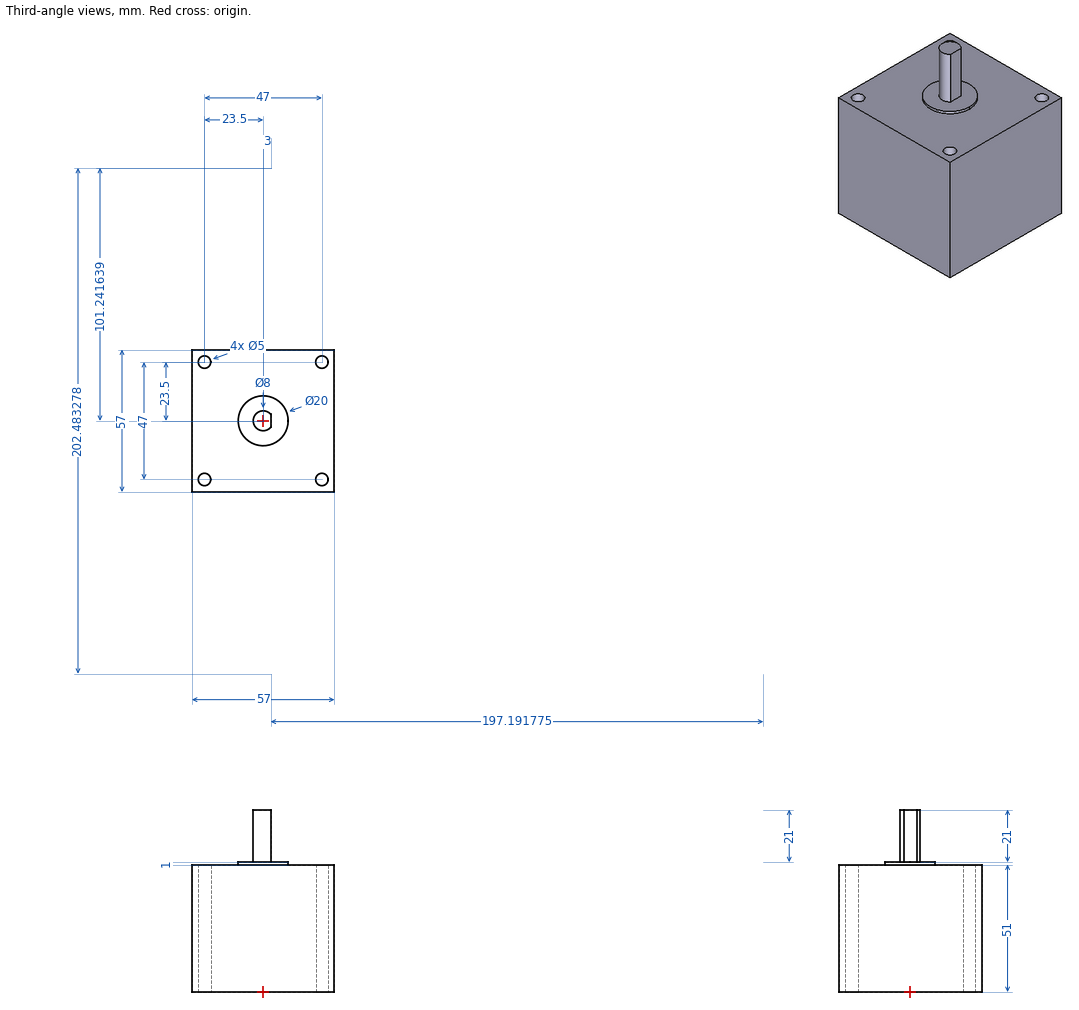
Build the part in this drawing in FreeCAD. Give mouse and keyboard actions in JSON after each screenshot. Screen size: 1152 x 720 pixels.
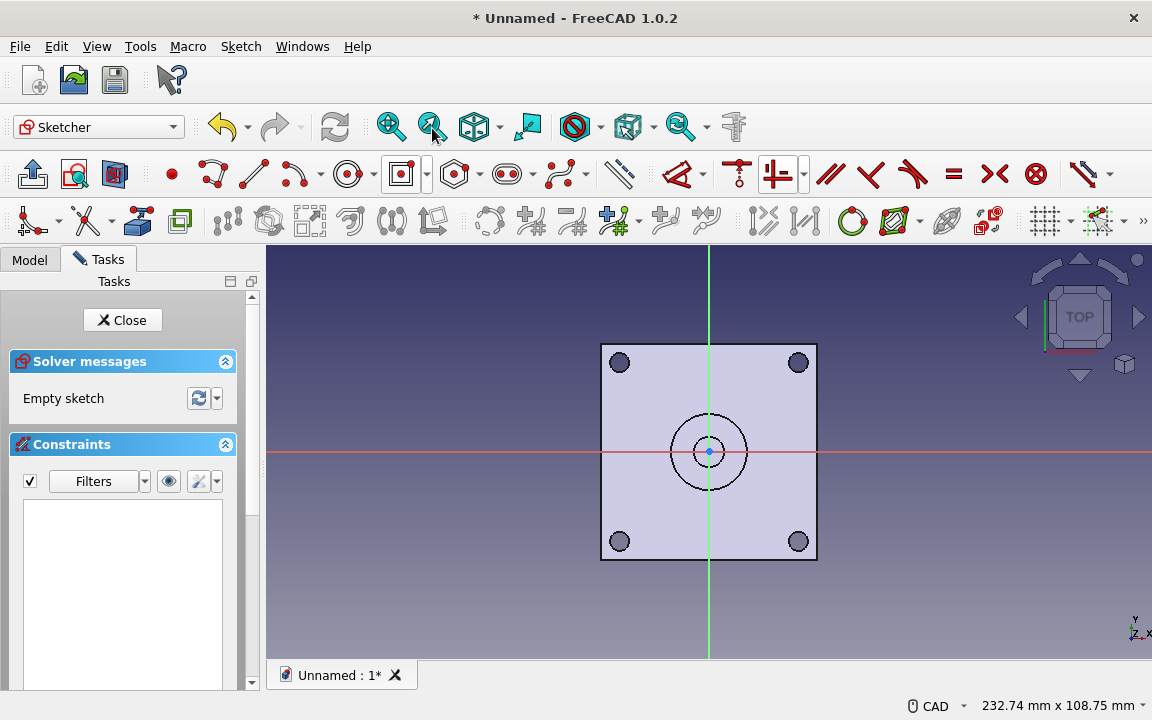
{"action": "scroll", "coordinate": [447, 452], "scroll_direction": "down", "scroll_amount": 6}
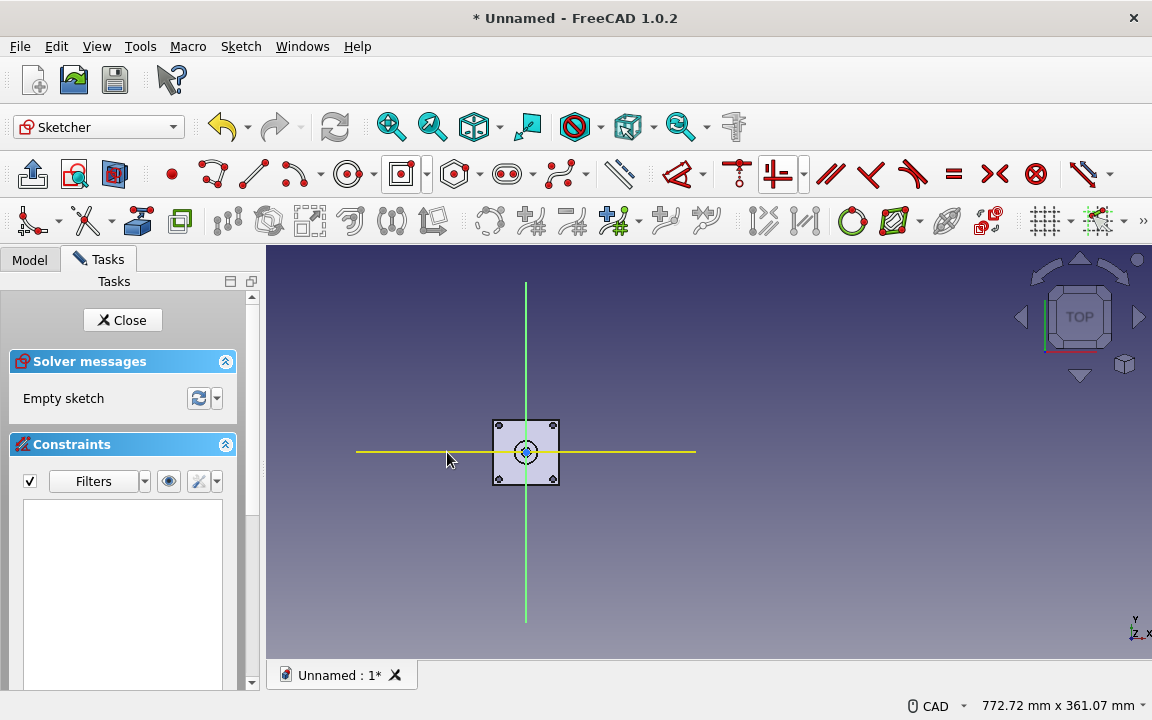
{"action": "left_click", "coordinate": [426, 174]}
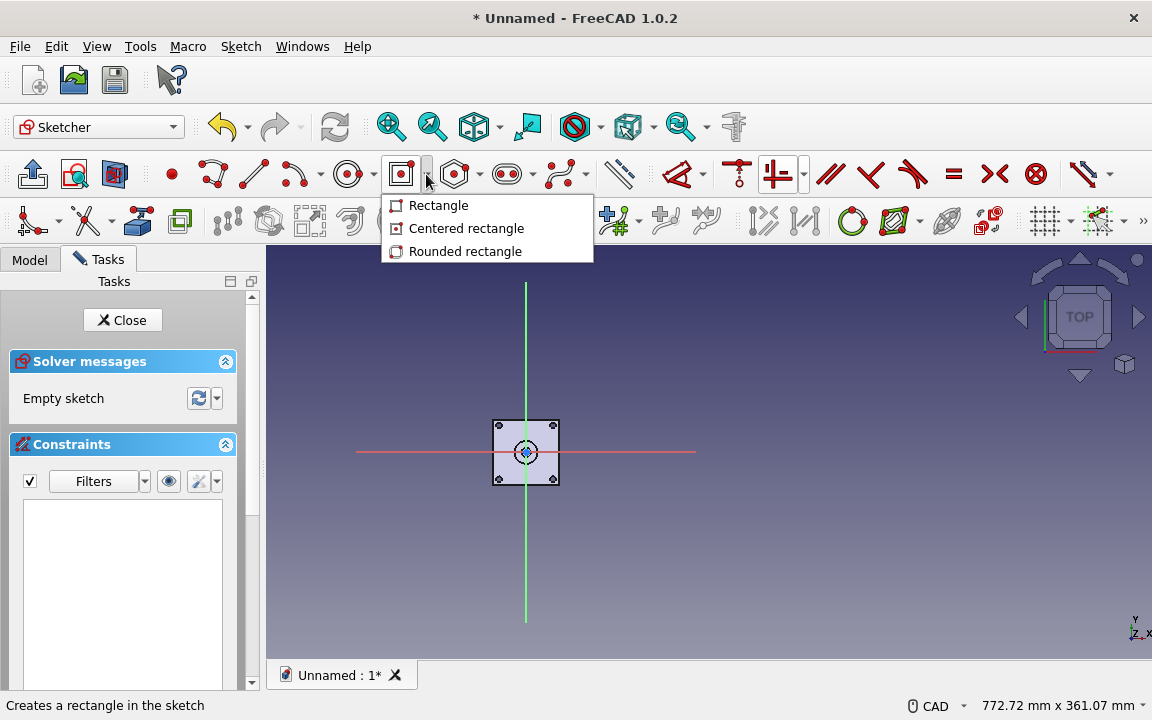
{"action": "left_click", "coordinate": [488, 206]}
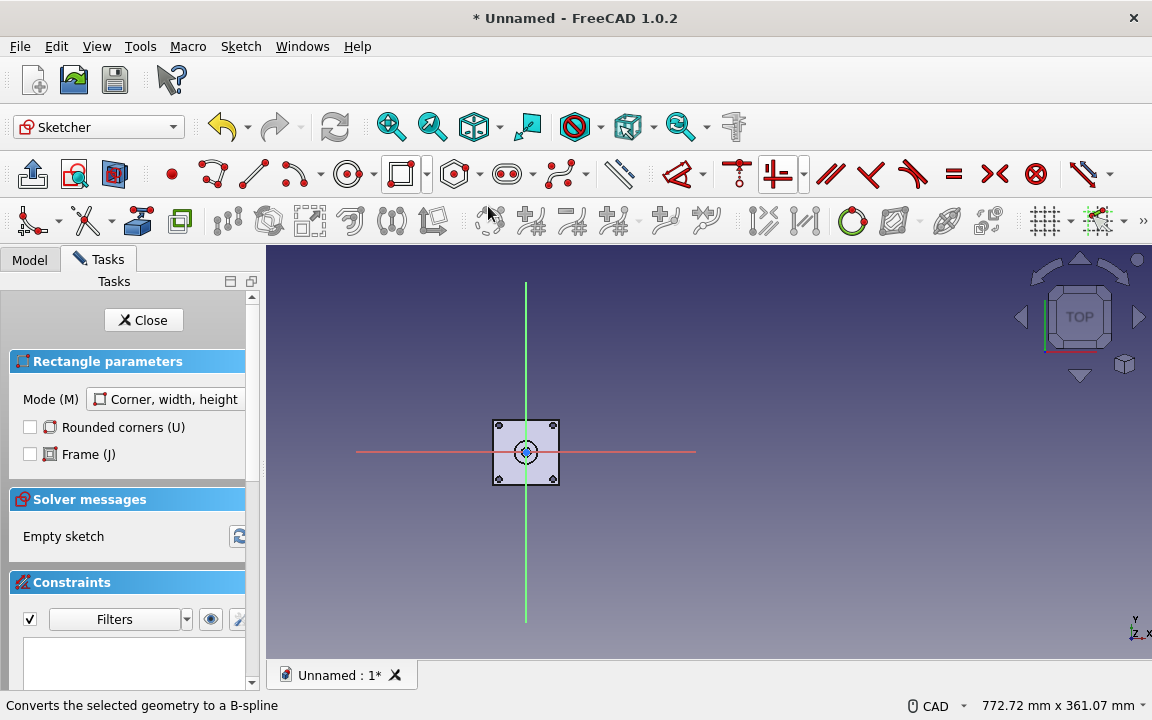
{"action": "scroll", "coordinate": [529, 336], "scroll_direction": "up", "scroll_amount": 8}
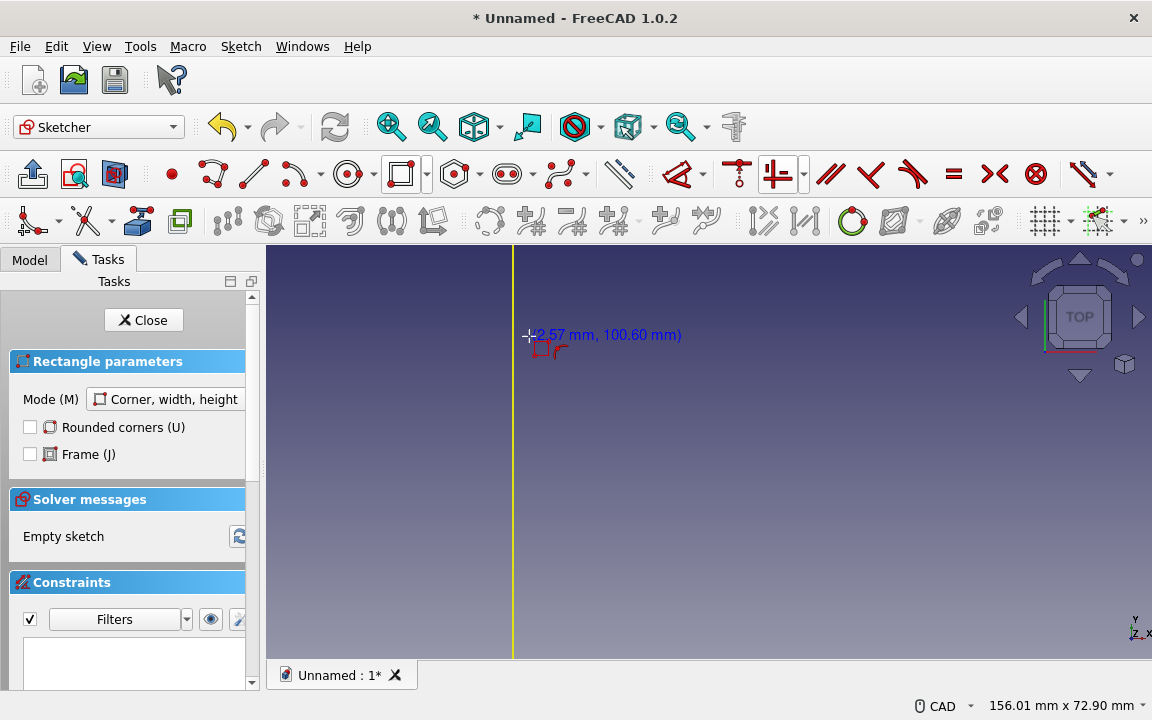
{"action": "left_click", "coordinate": [530, 336]}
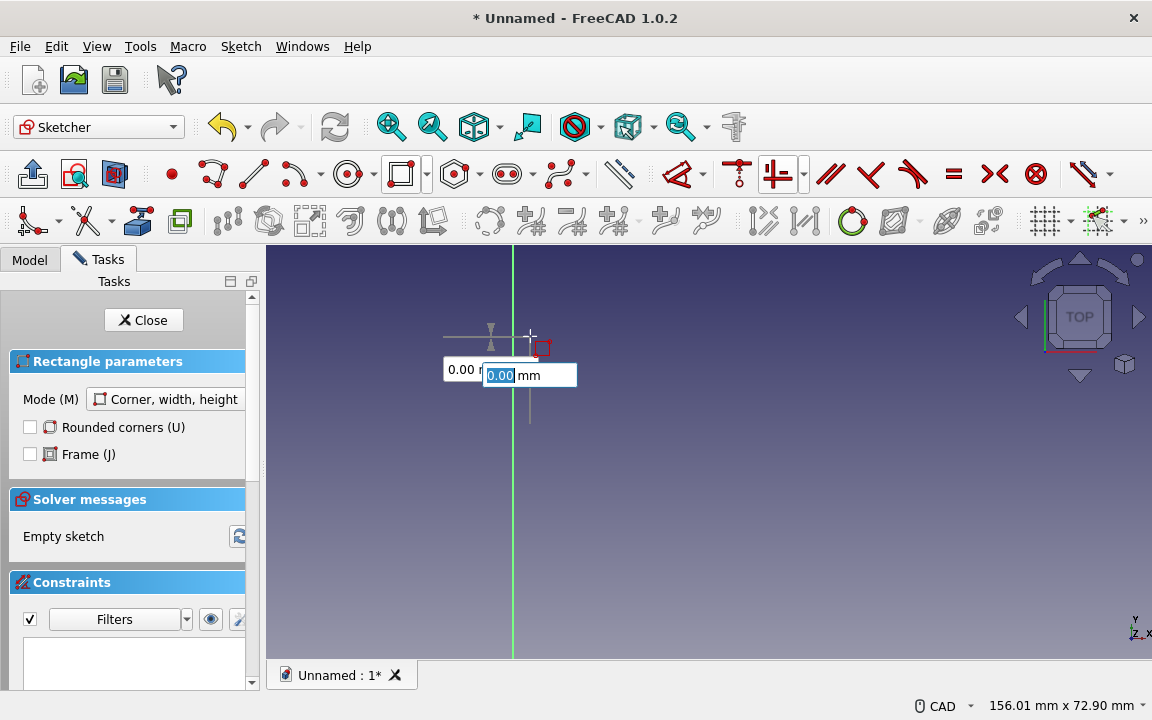
{"action": "scroll", "coordinate": [529, 336], "scroll_direction": "down", "scroll_amount": 8}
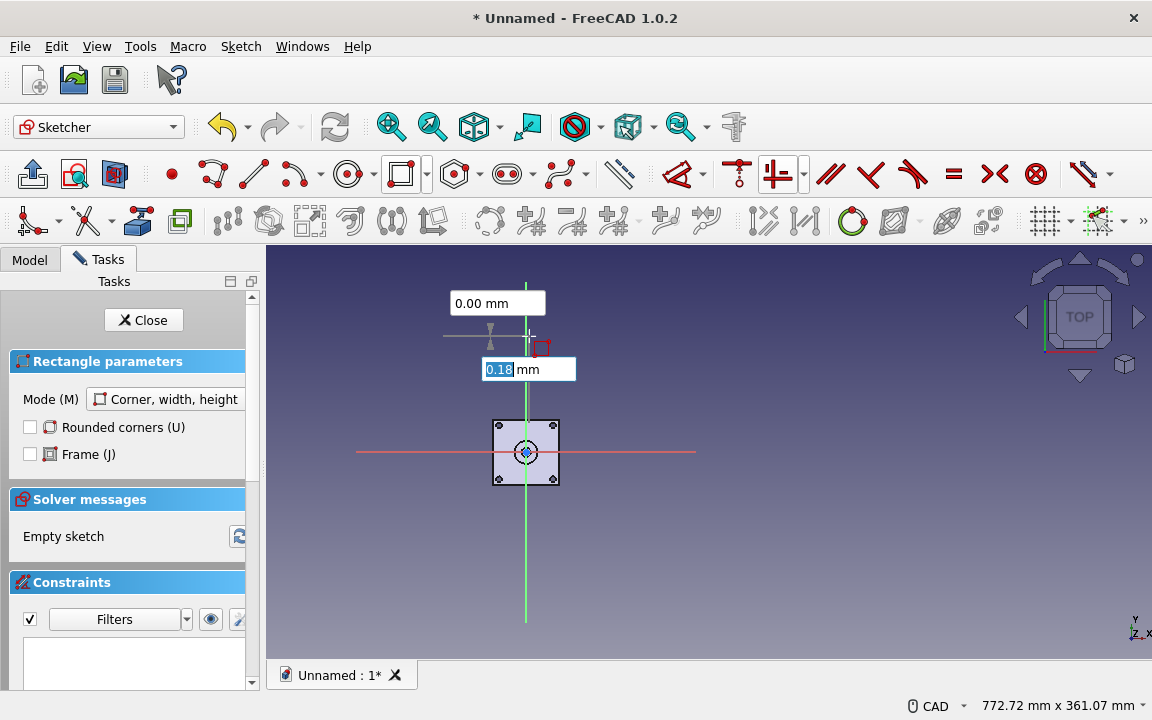
{"action": "left_click", "coordinate": [756, 568]}
{"action": "key", "text": "Escape"}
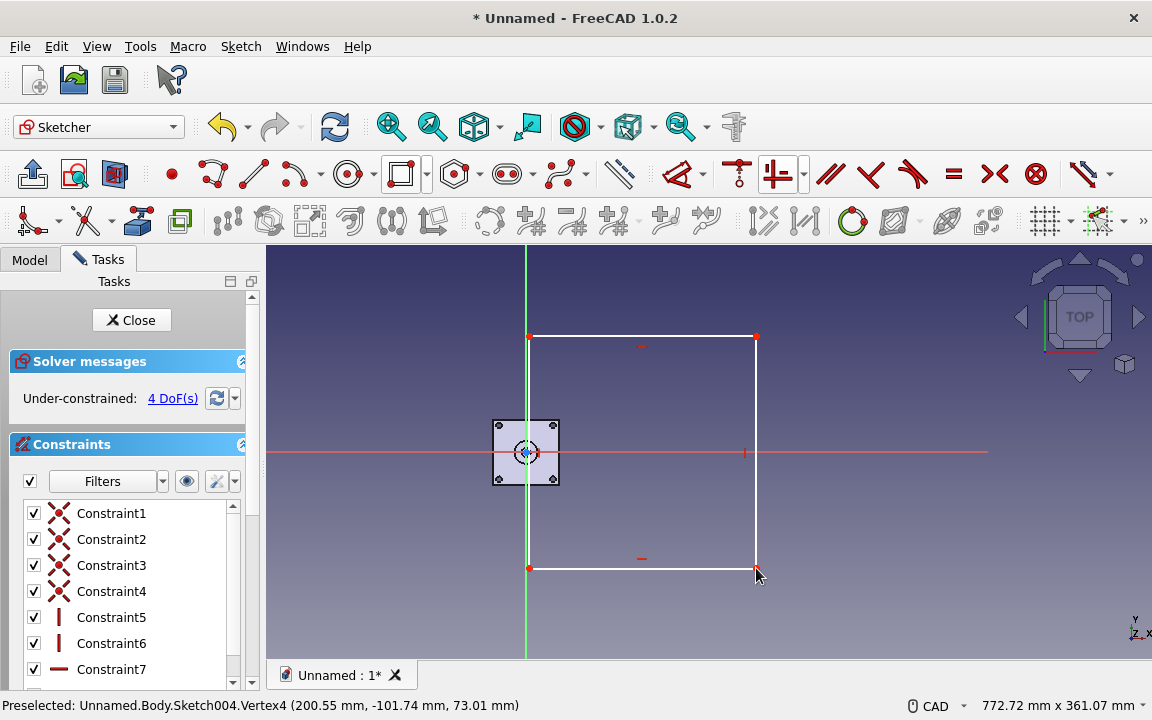
{"action": "left_click", "coordinate": [676, 174]}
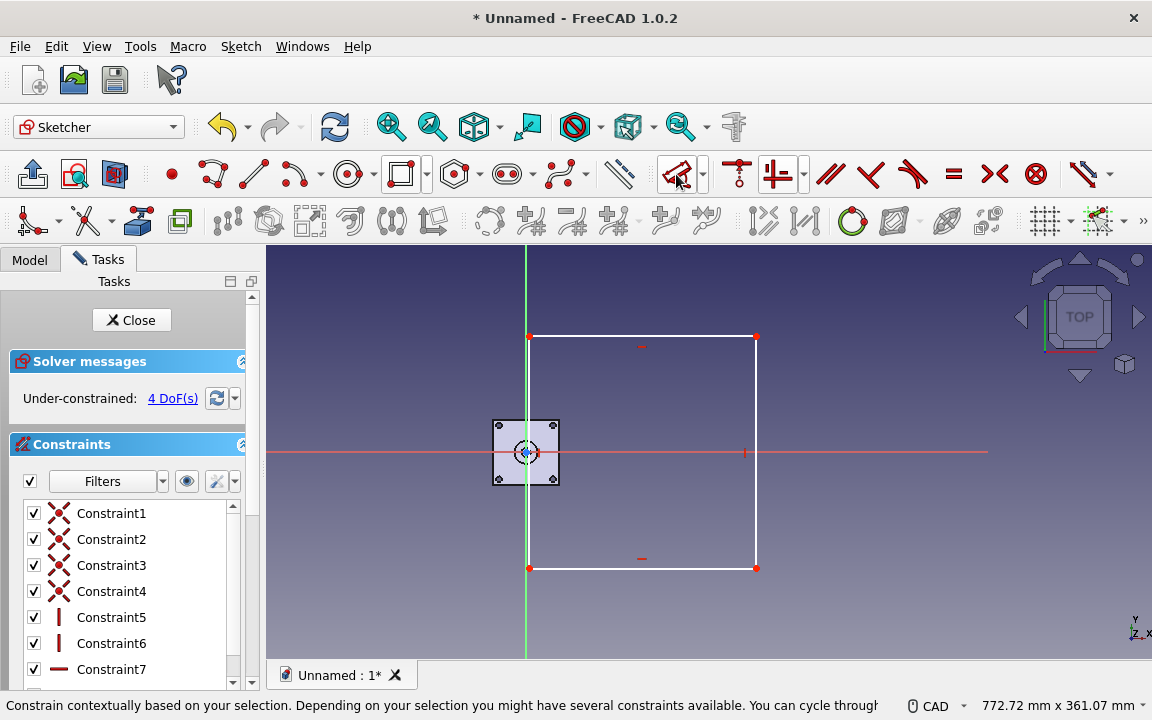
{"action": "scroll", "coordinate": [529, 336], "scroll_direction": "up", "scroll_amount": 13}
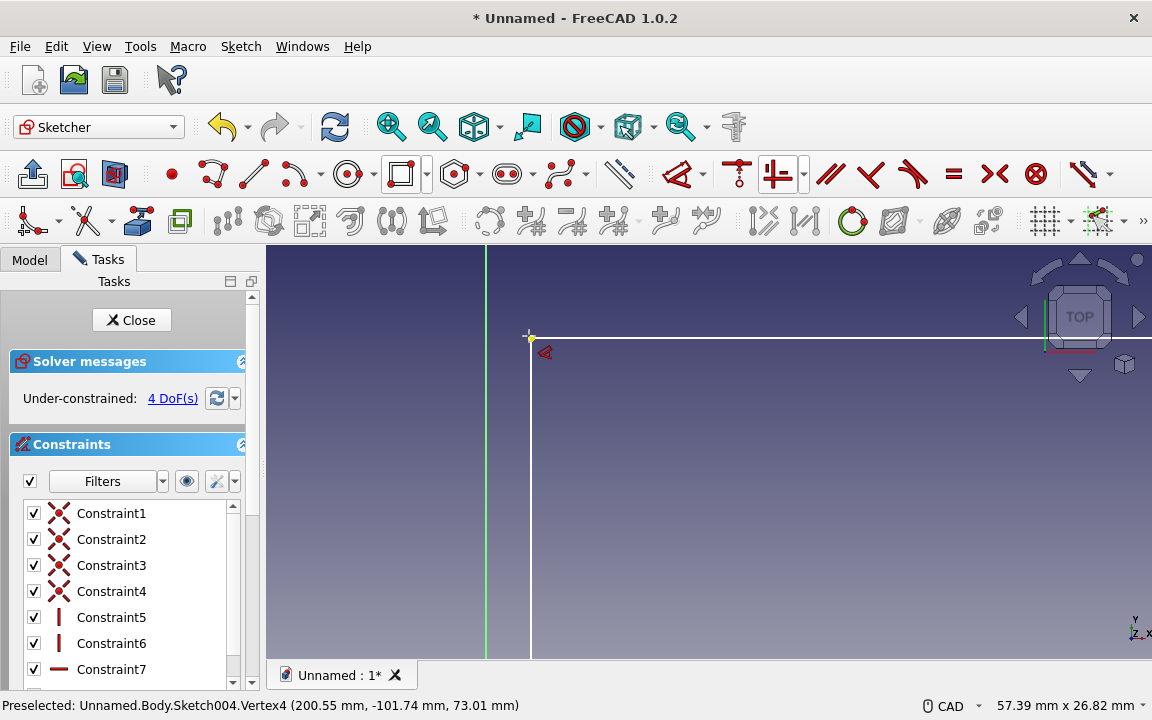
{"action": "left_click", "coordinate": [531, 338]}
{"action": "left_click", "coordinate": [508, 304]}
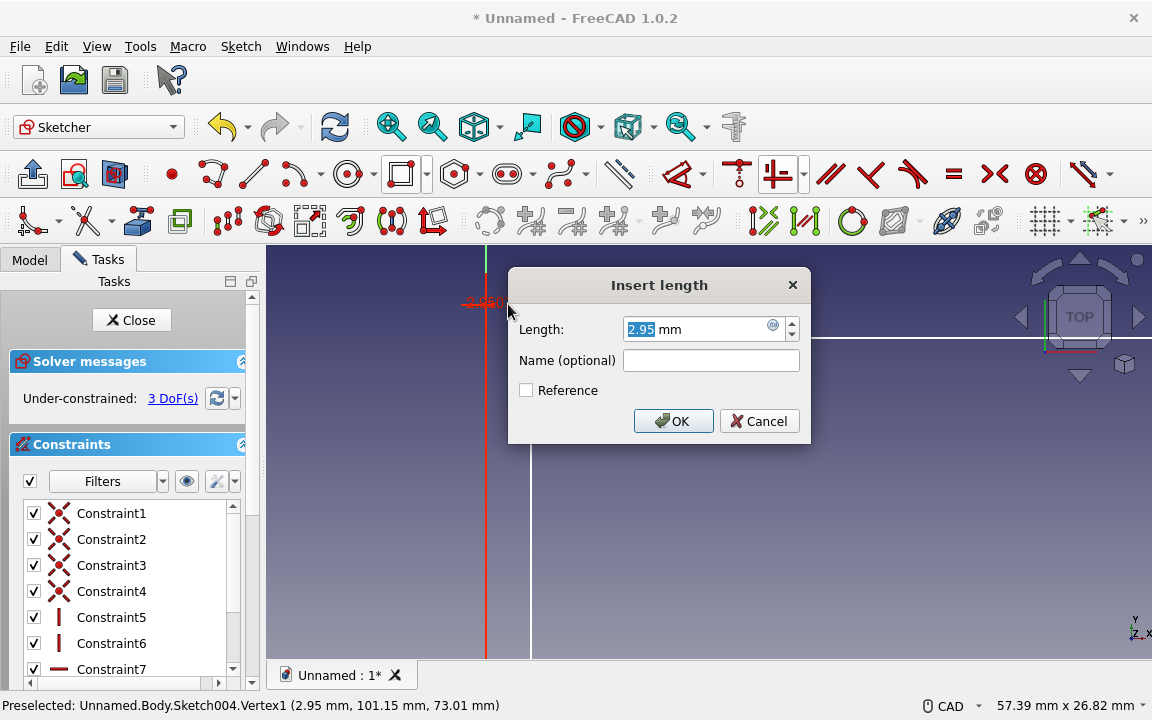
{"action": "type", "text": "3"}
{"action": "key", "text": "Return"}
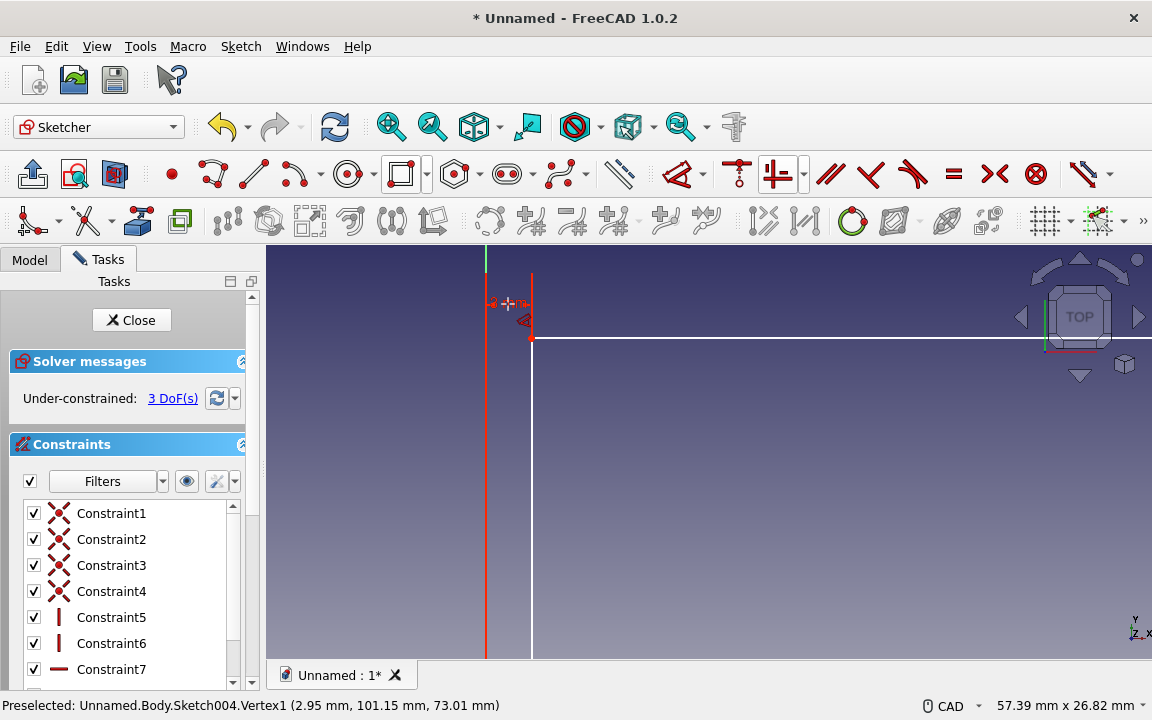
{"action": "scroll", "coordinate": [529, 336], "scroll_direction": "down", "scroll_amount": 13}